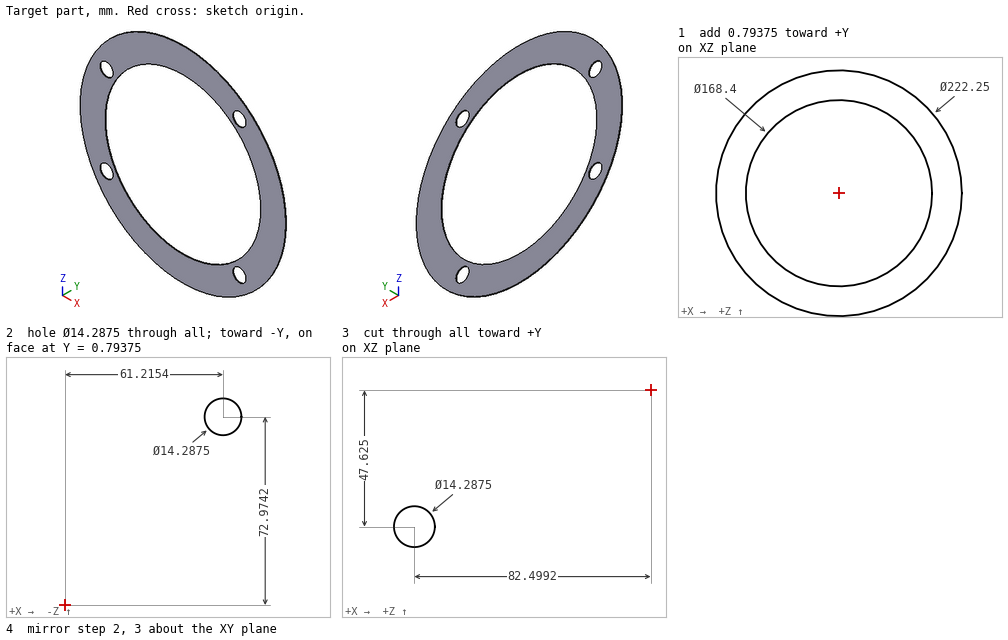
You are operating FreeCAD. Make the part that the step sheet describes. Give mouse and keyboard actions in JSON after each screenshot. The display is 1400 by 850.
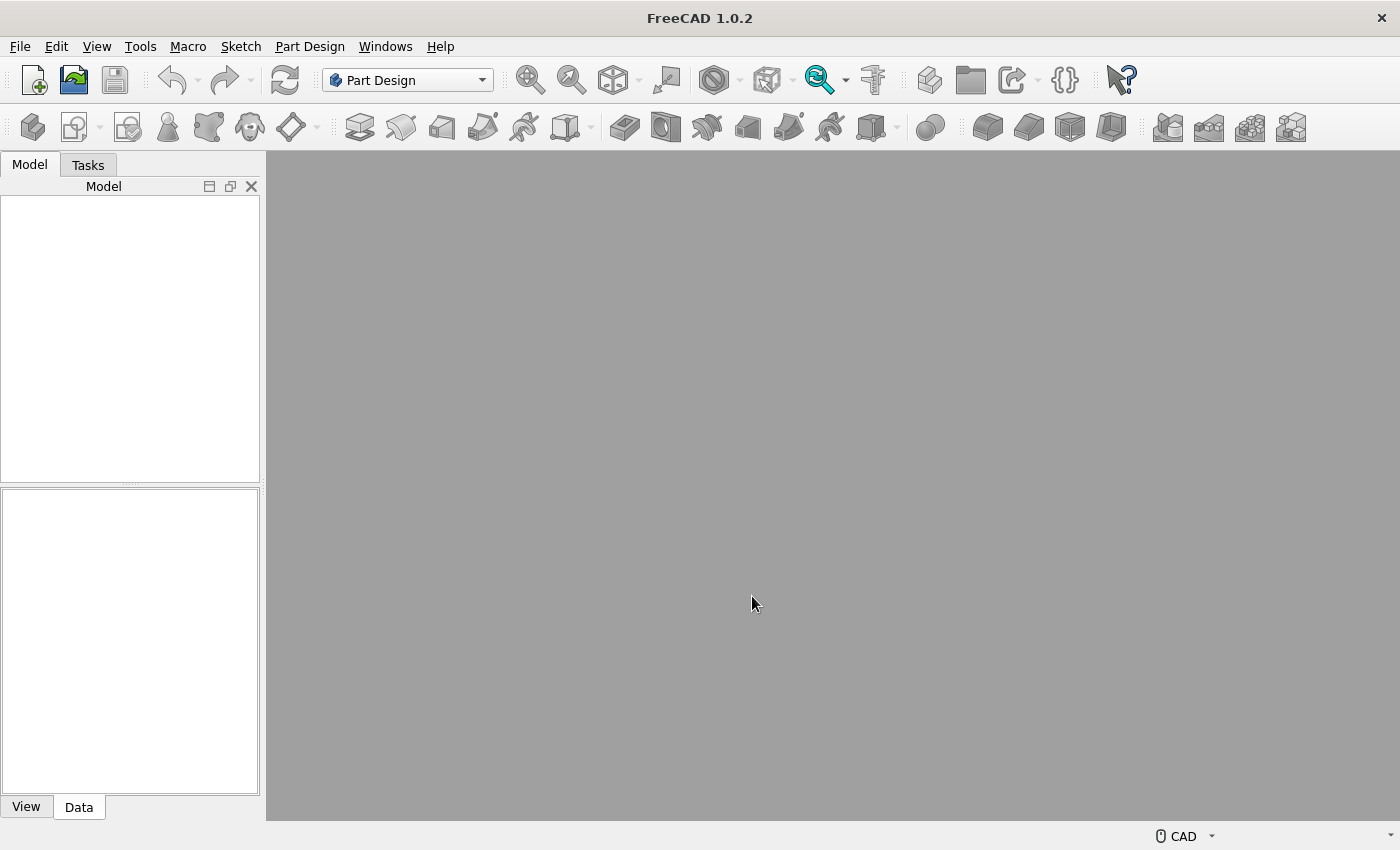
{"action": "left_click", "coordinate": [33, 80]}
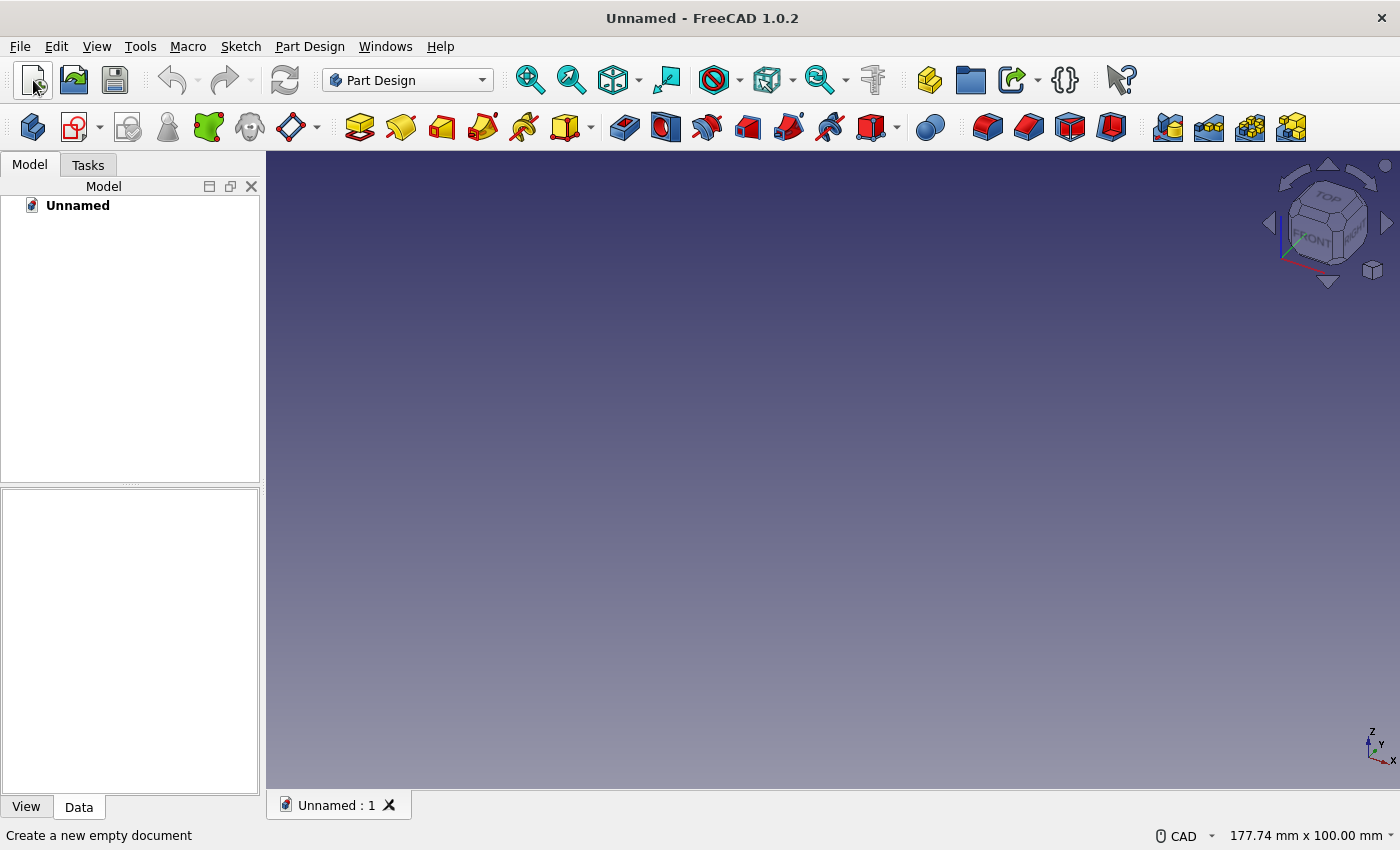
{"action": "left_click", "coordinate": [74, 128]}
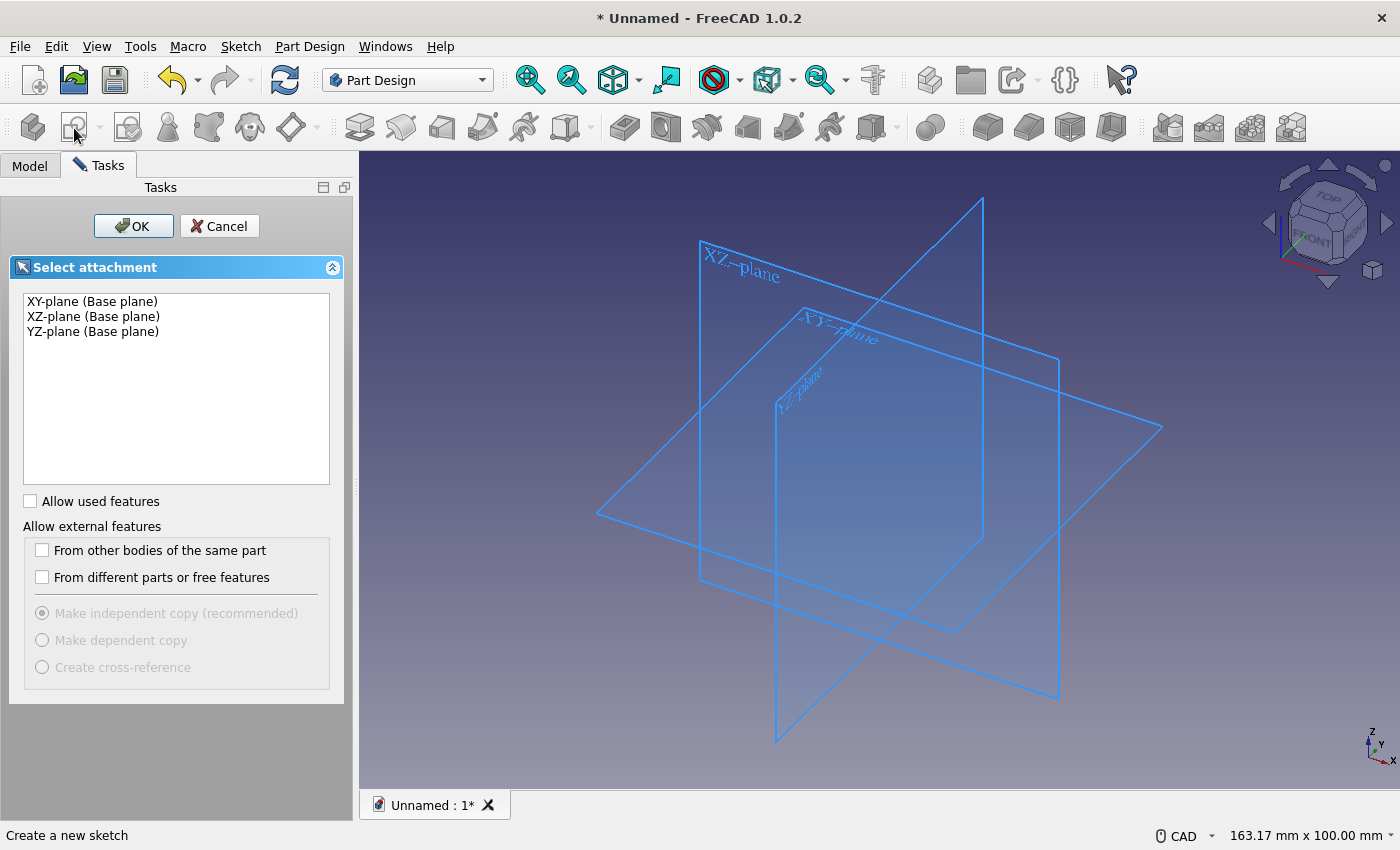
{"action": "left_click", "coordinate": [84, 316]}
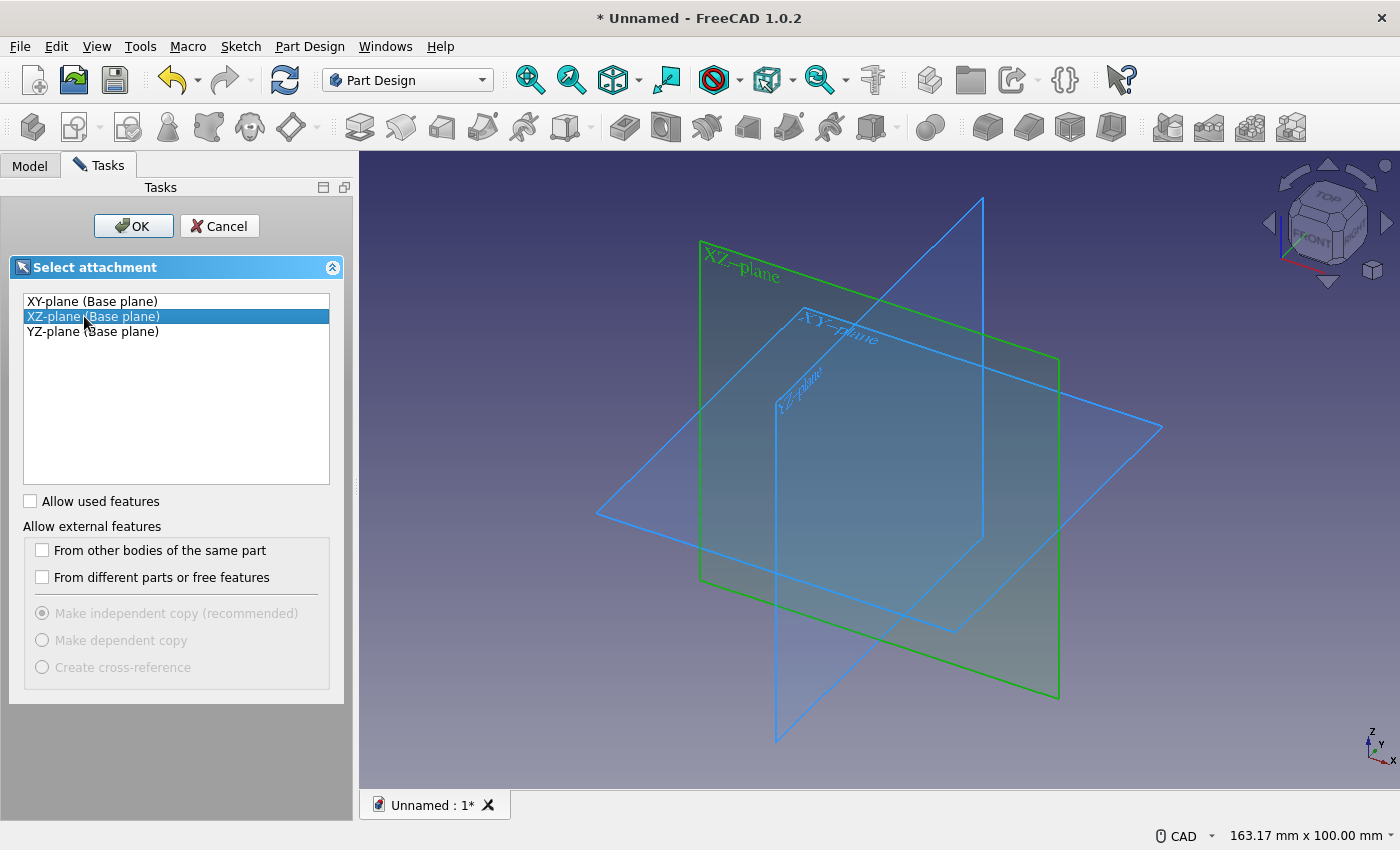
{"action": "left_click", "coordinate": [134, 226]}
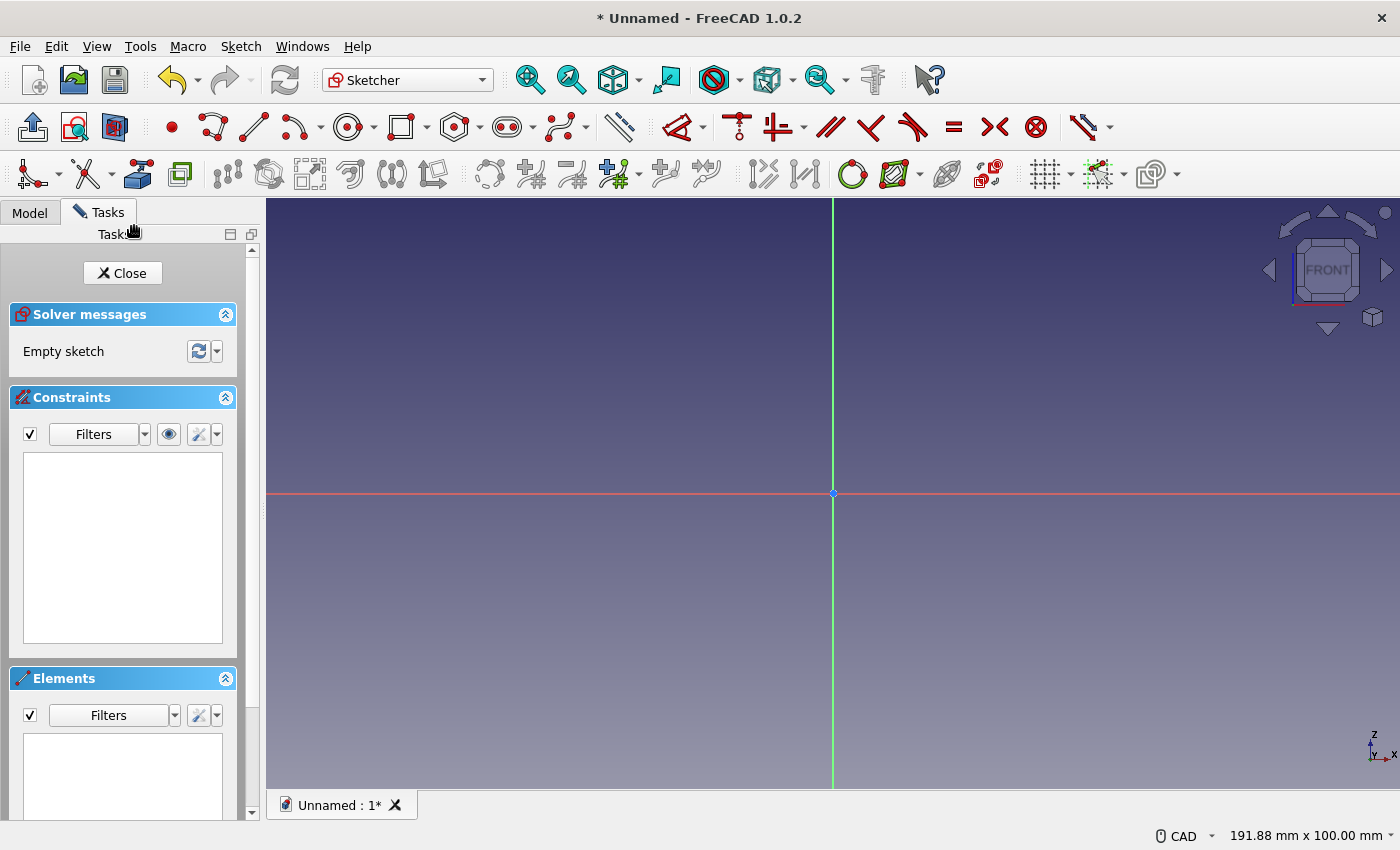
{"action": "scroll", "coordinate": [735, 493], "scroll_direction": "down", "scroll_amount": 6}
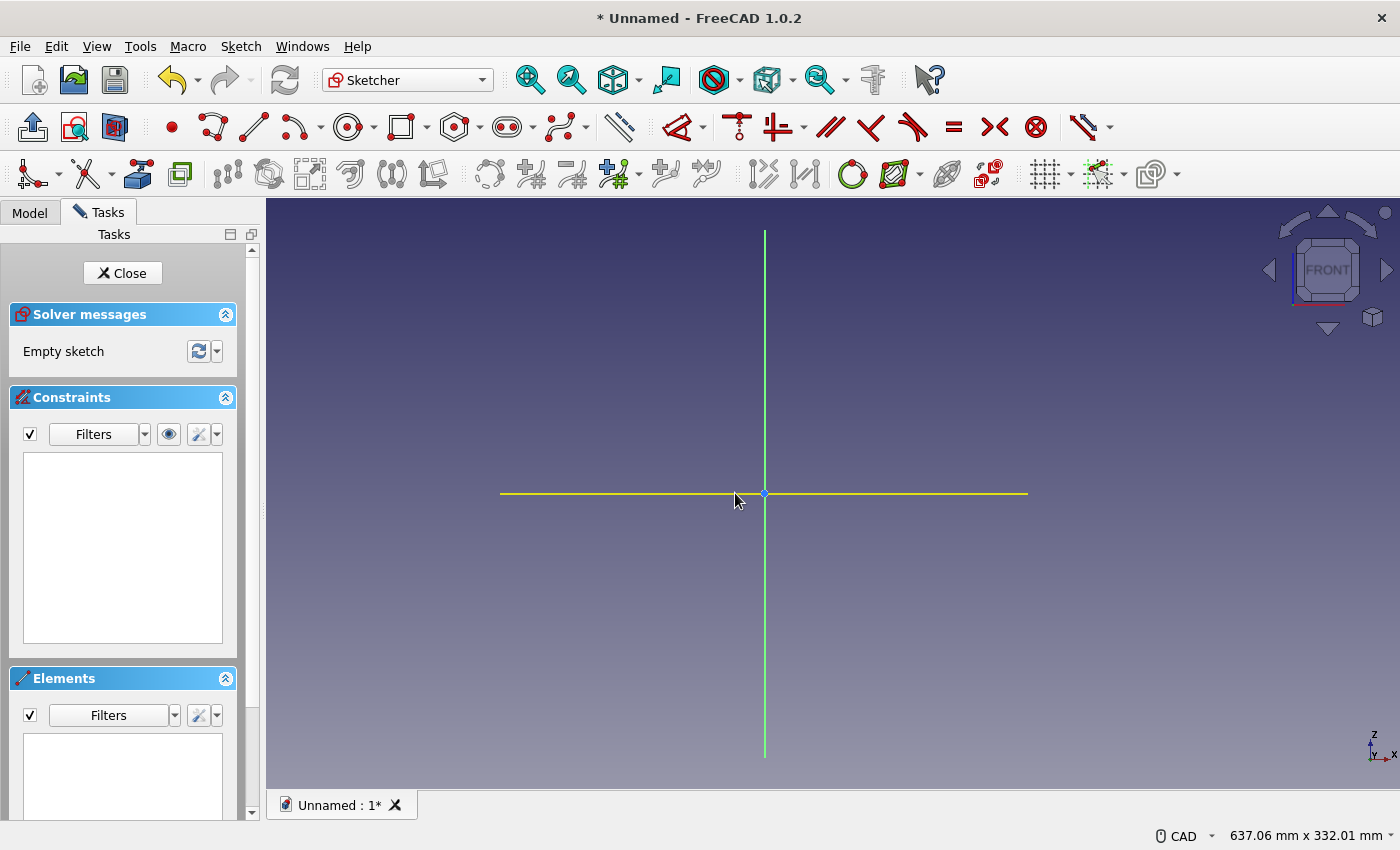
{"action": "left_click", "coordinate": [348, 128]}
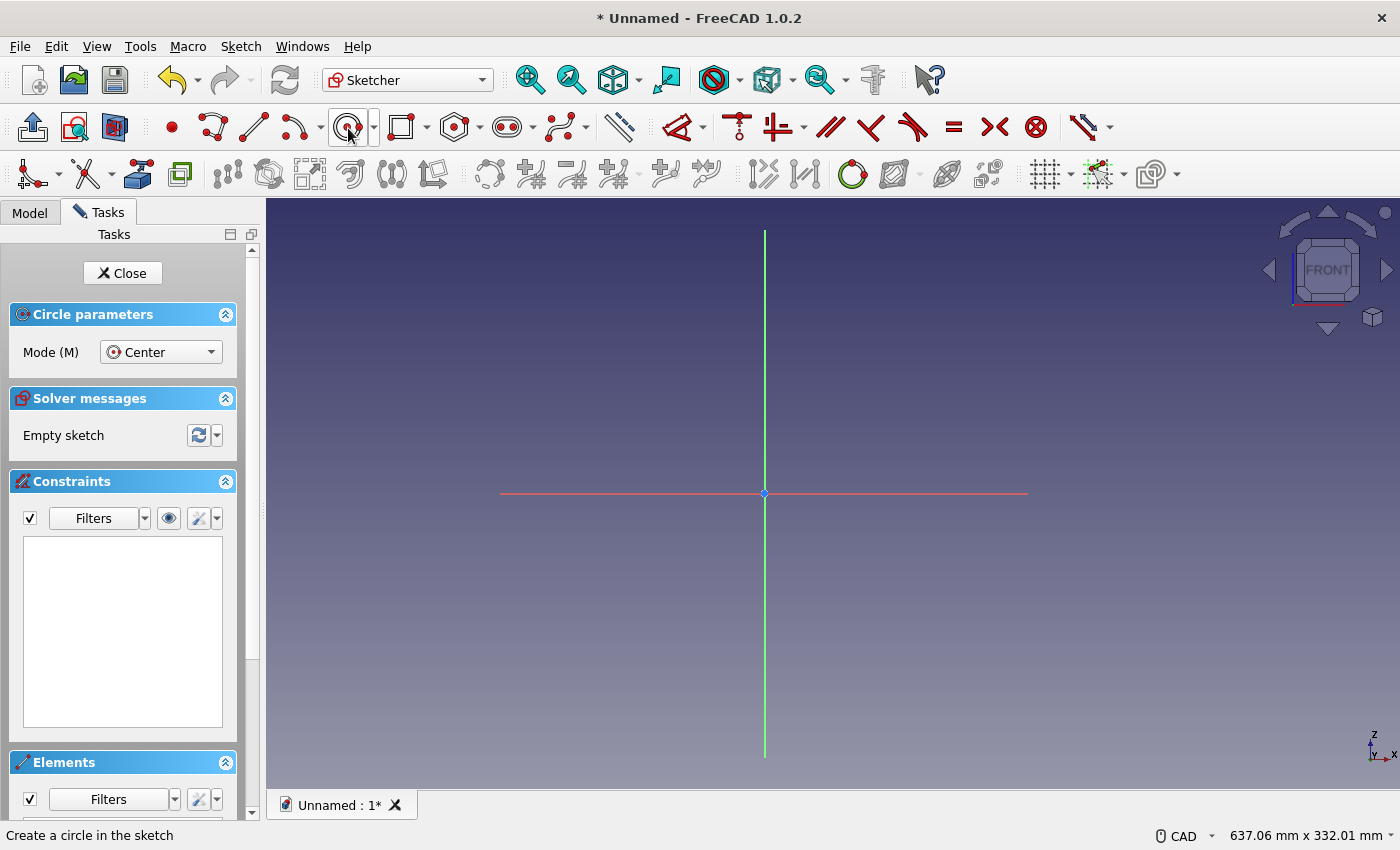
{"action": "left_click", "coordinate": [765, 494]}
{"action": "left_click", "coordinate": [905, 354]}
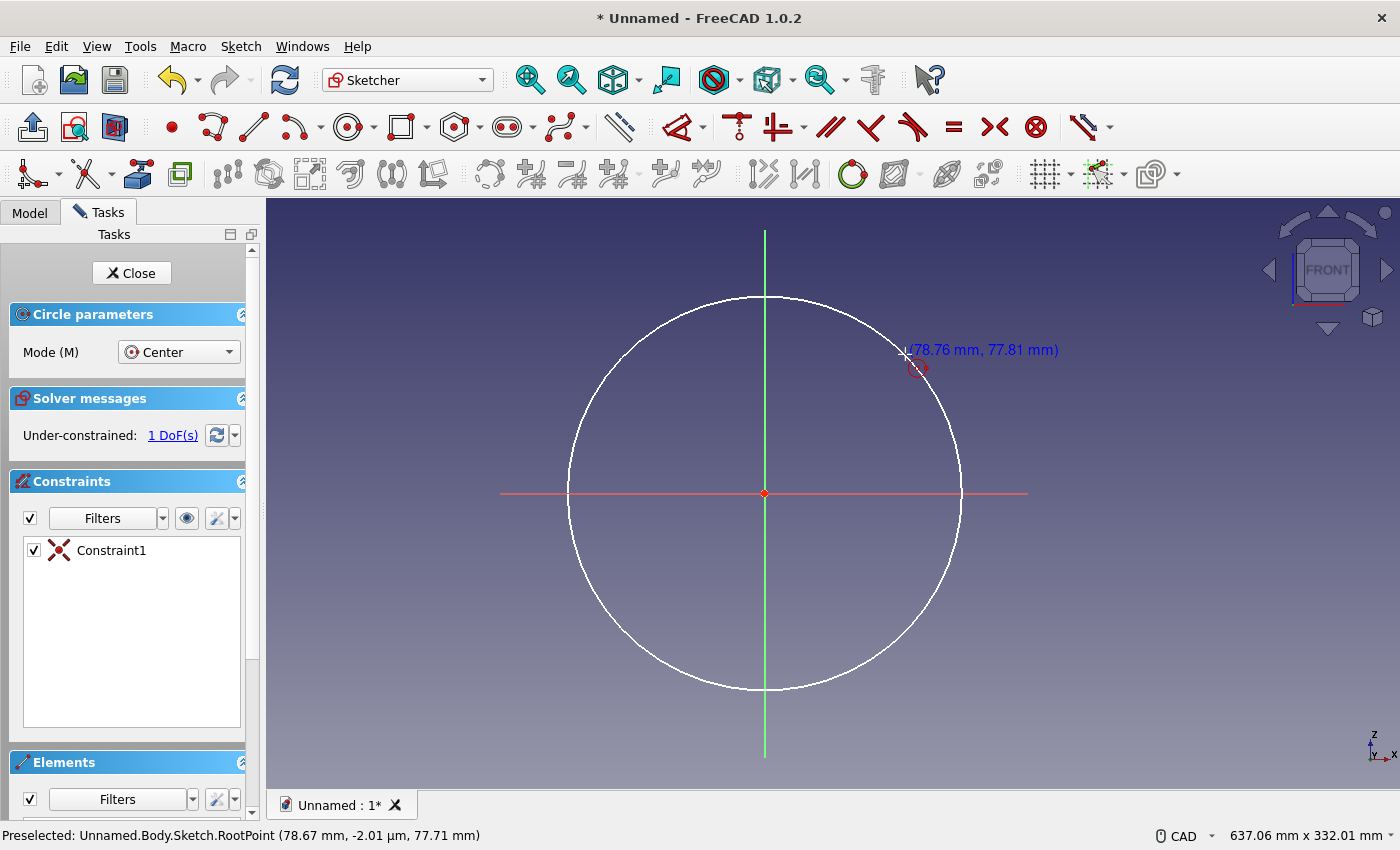
{"action": "left_click", "coordinate": [765, 494]}
{"action": "left_click", "coordinate": [871, 388]}
{"action": "key", "text": "Escape"}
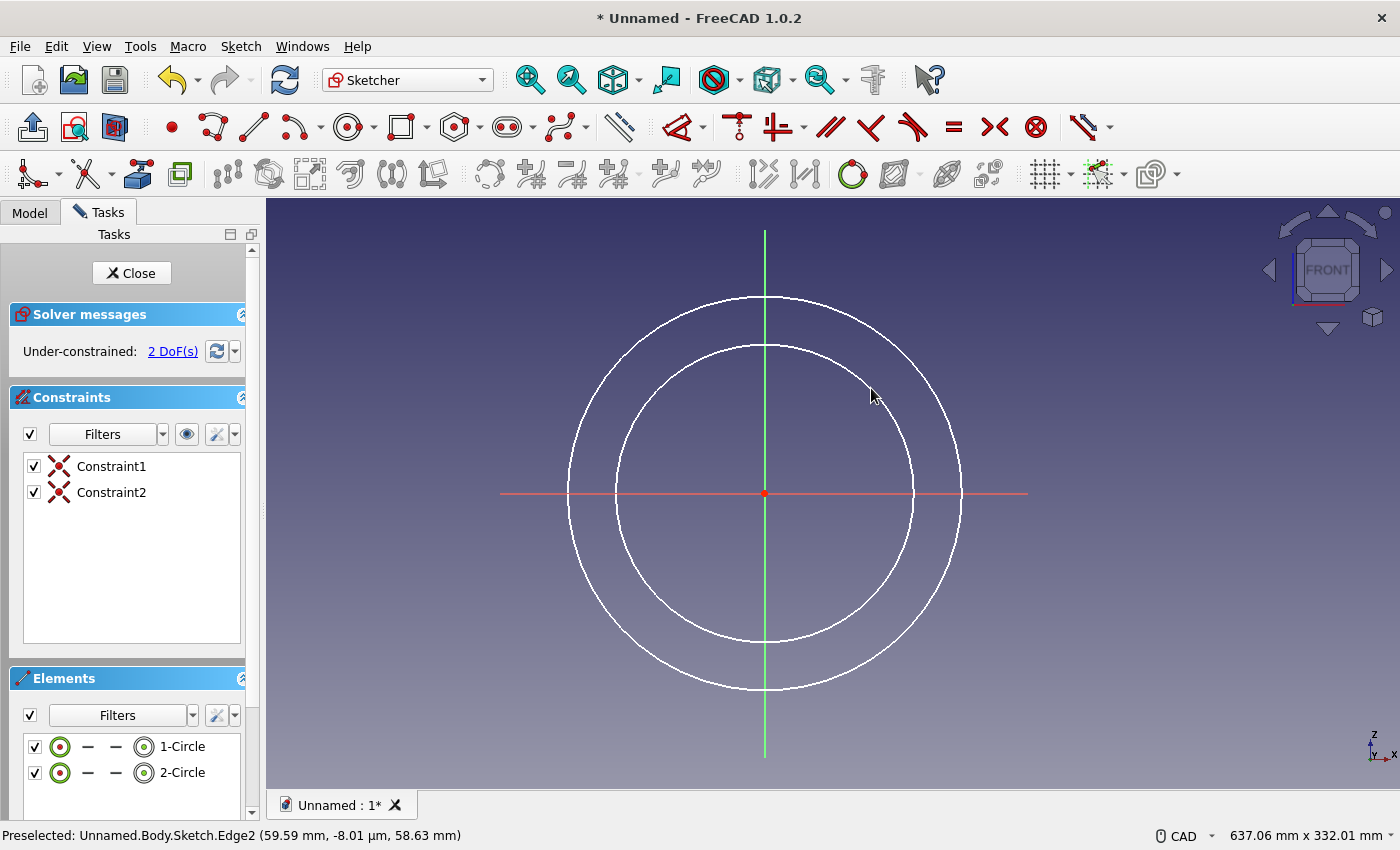
{"action": "left_click", "coordinate": [904, 354]}